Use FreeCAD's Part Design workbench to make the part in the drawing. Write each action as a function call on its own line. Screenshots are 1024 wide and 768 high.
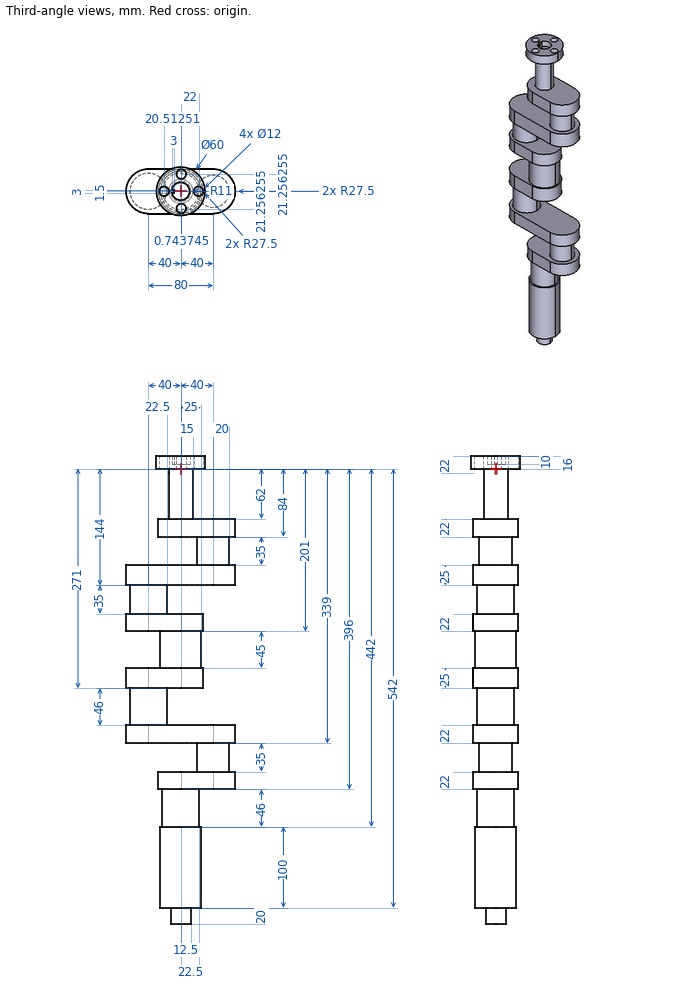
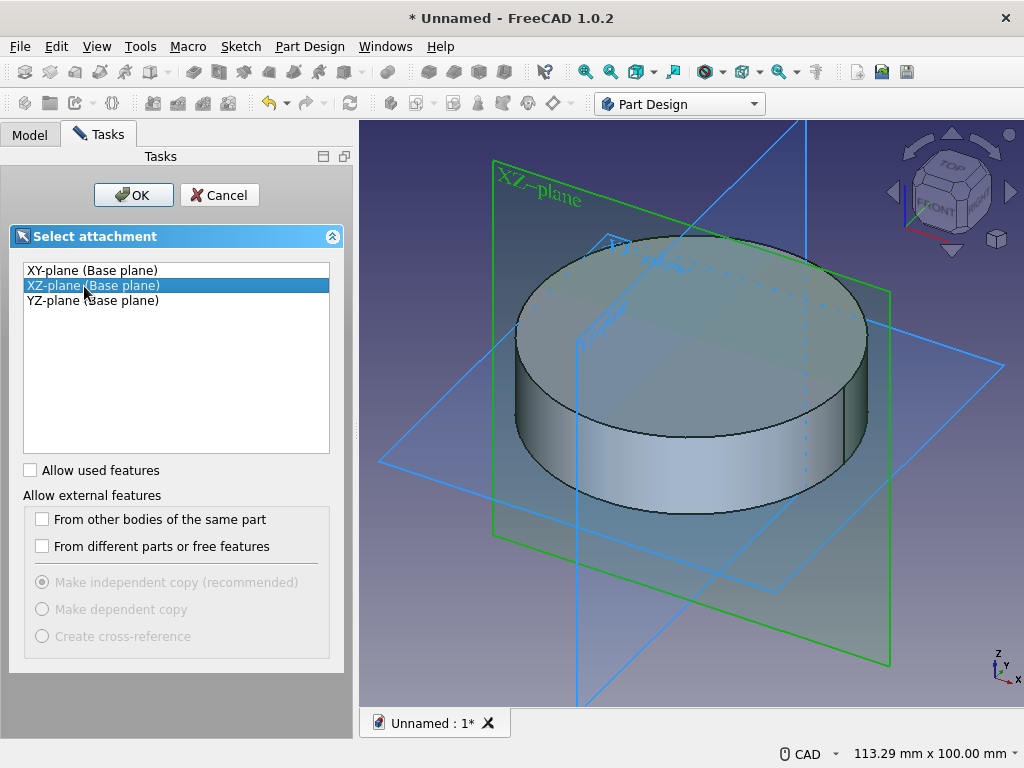
click(134, 195)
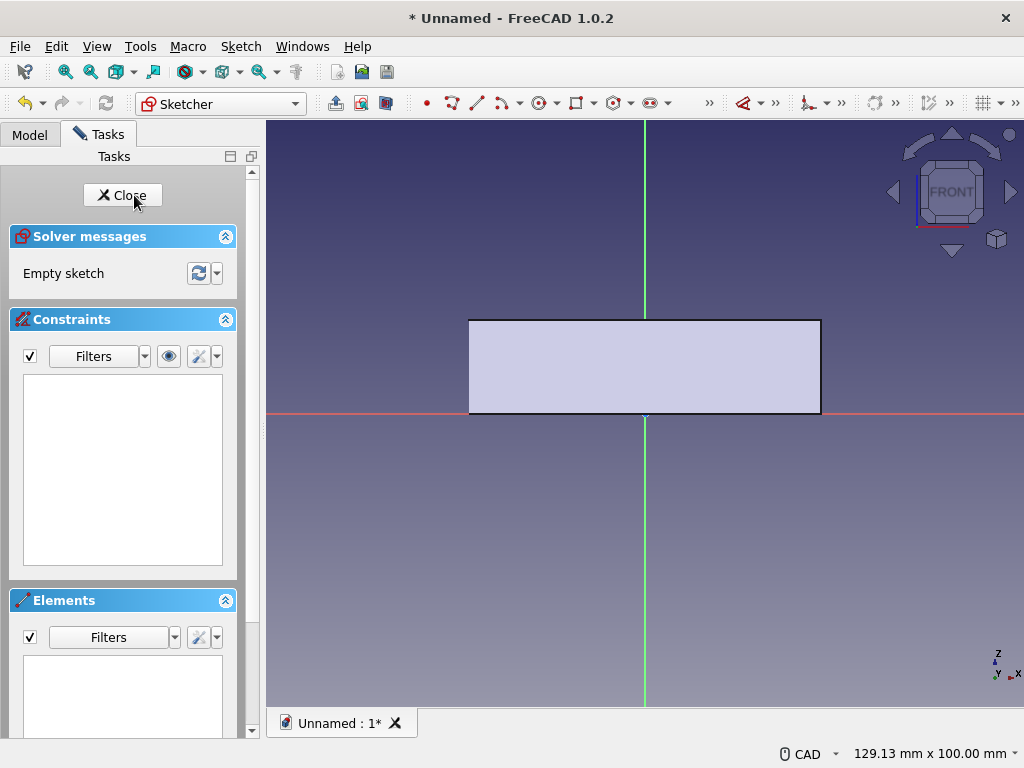
key(q)
key(s)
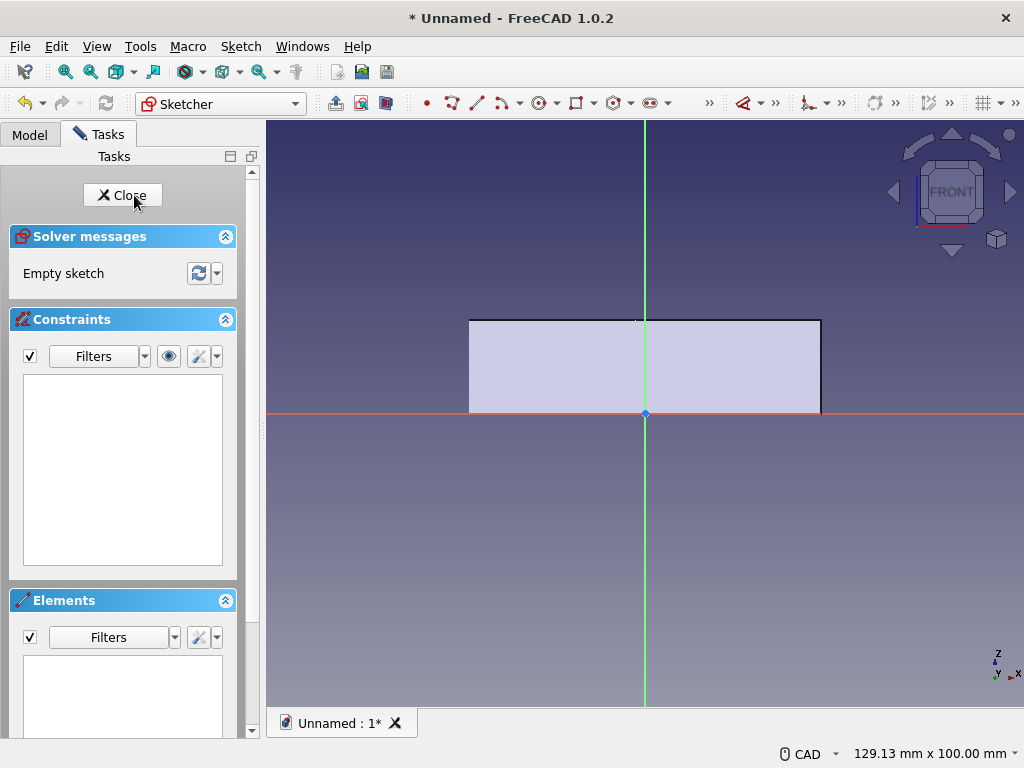
scroll(348, 148, down, 2)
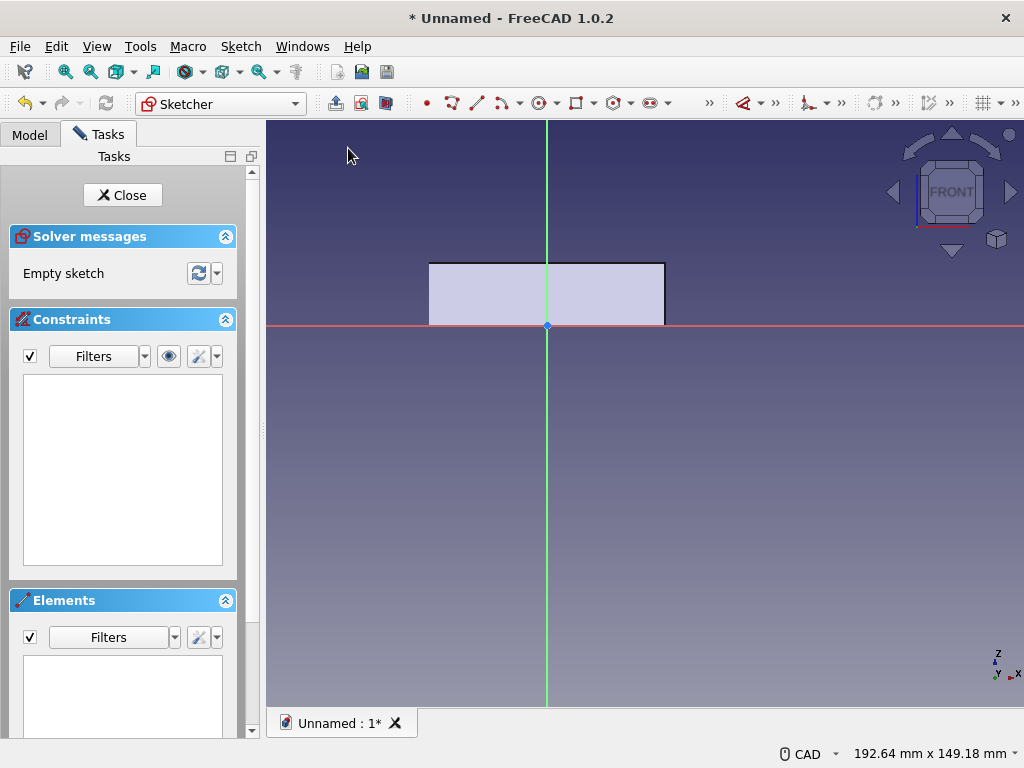
scroll(577, 518, up, 2)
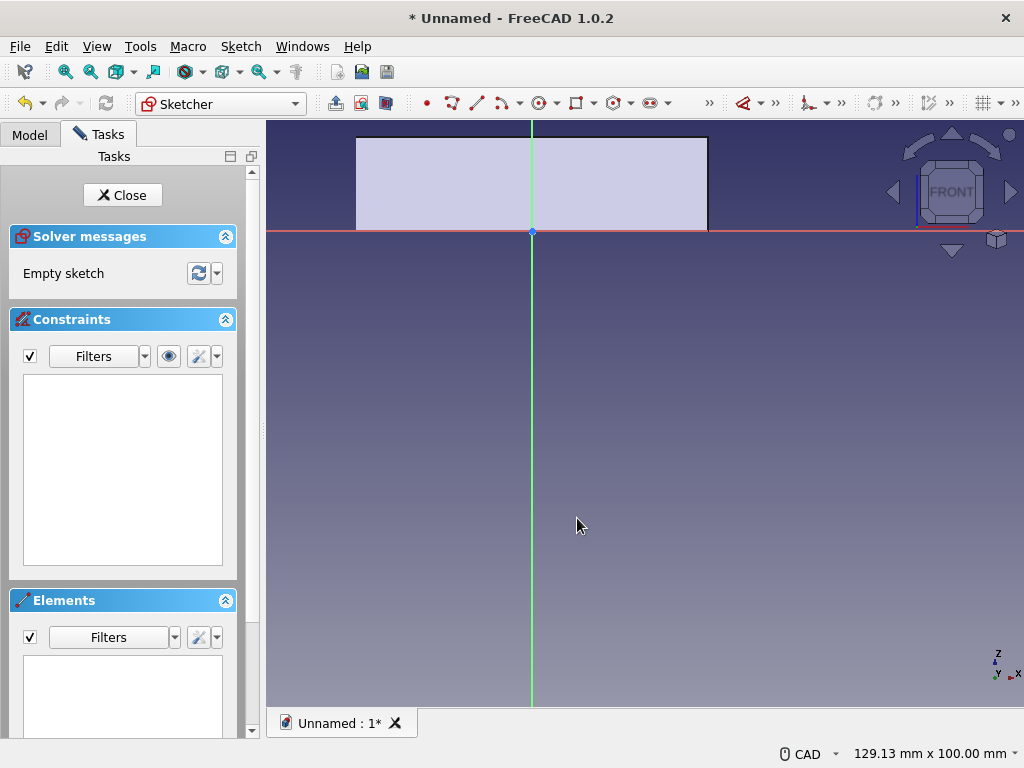
click(576, 104)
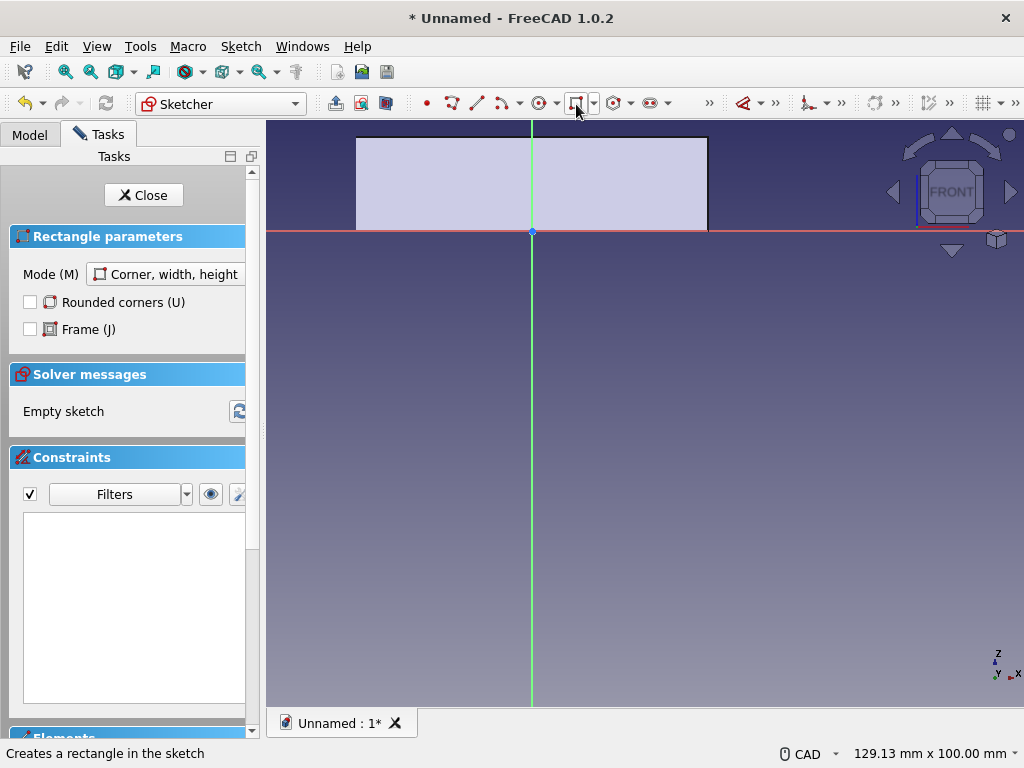
click(532, 231)
move(620, 595)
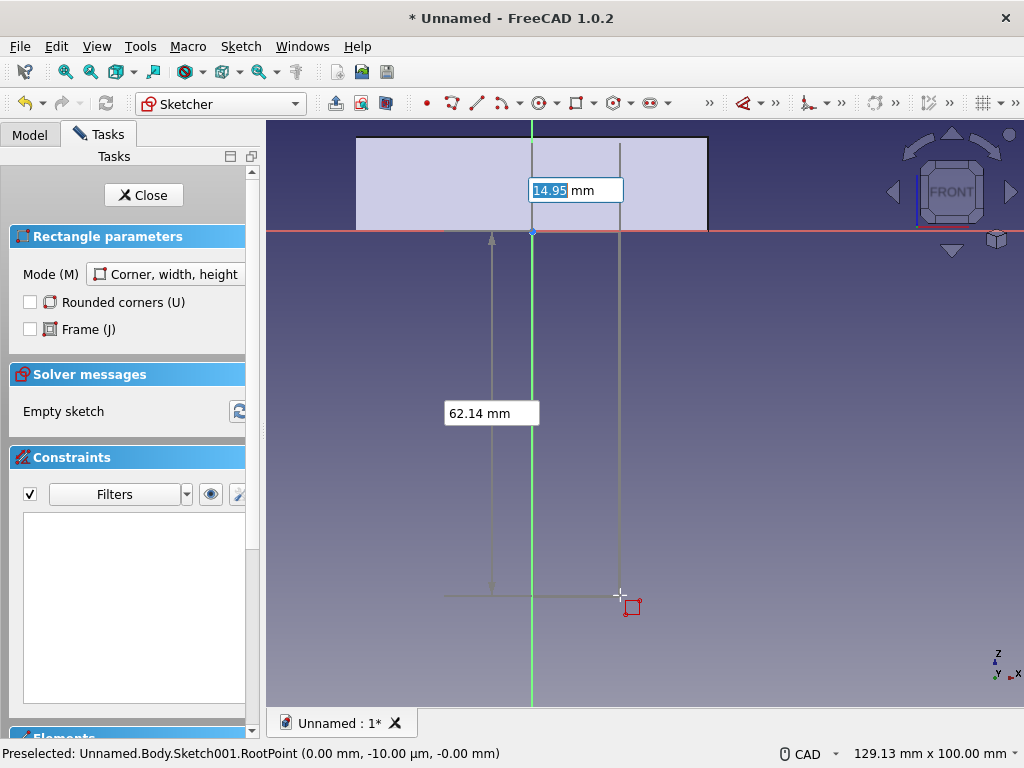
text(15)
key(Tab)
text(62)
key(Return)
key(Escape)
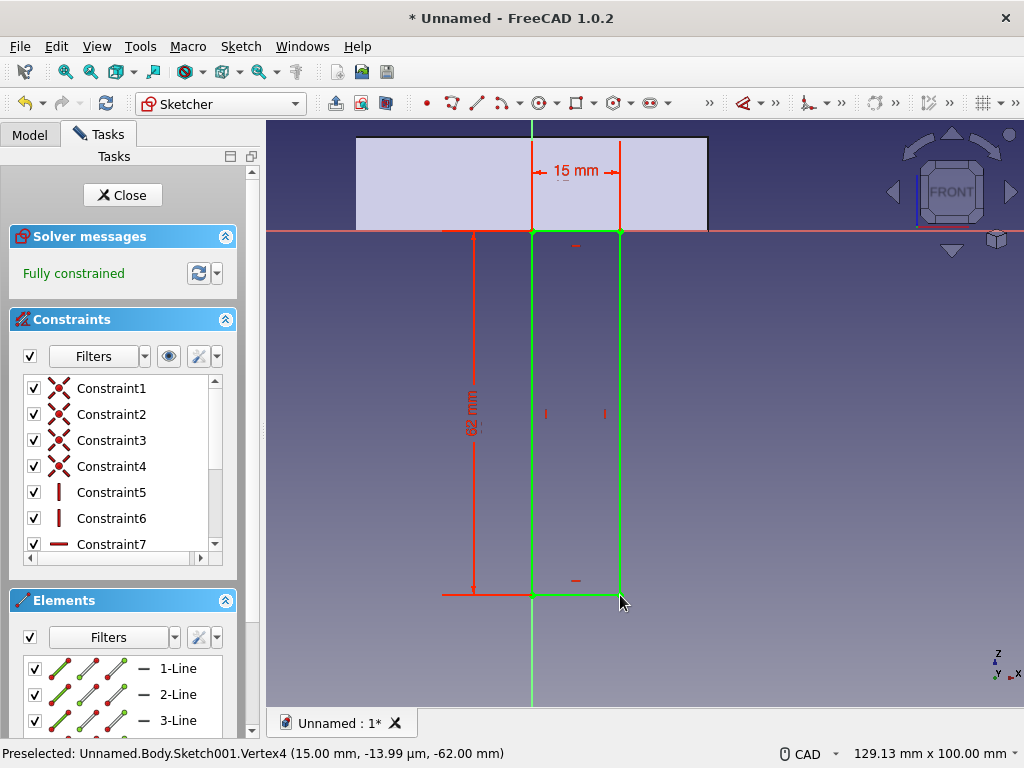
click(123, 195)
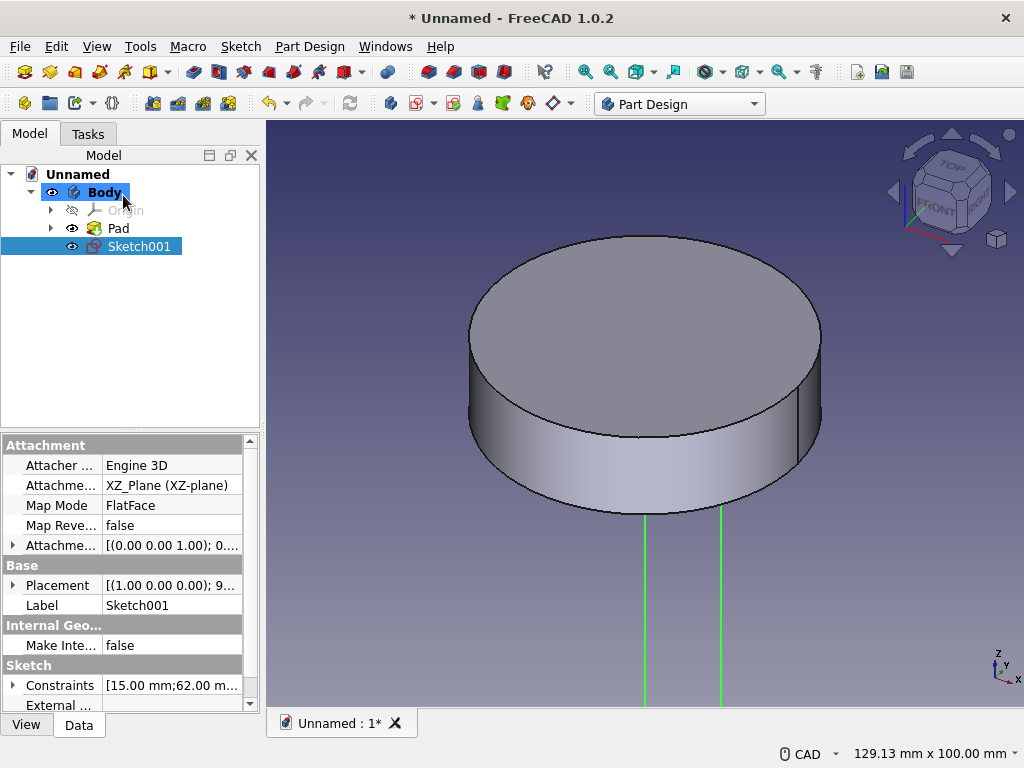
click(50, 72)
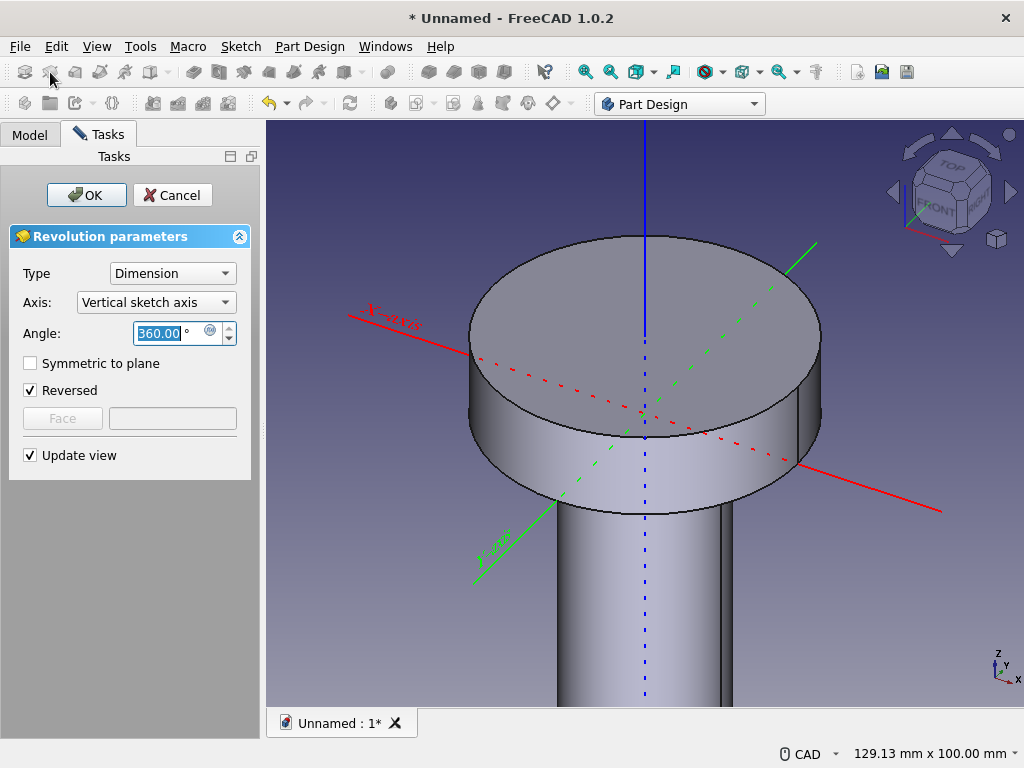
click(87, 195)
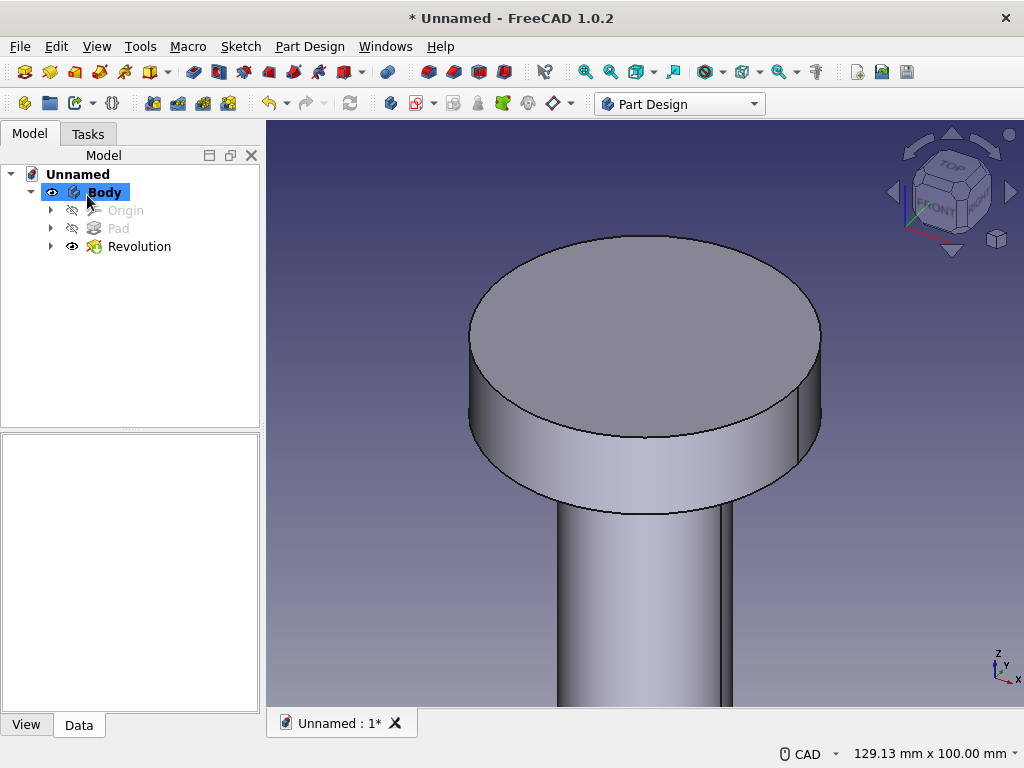
key(v)
key(f)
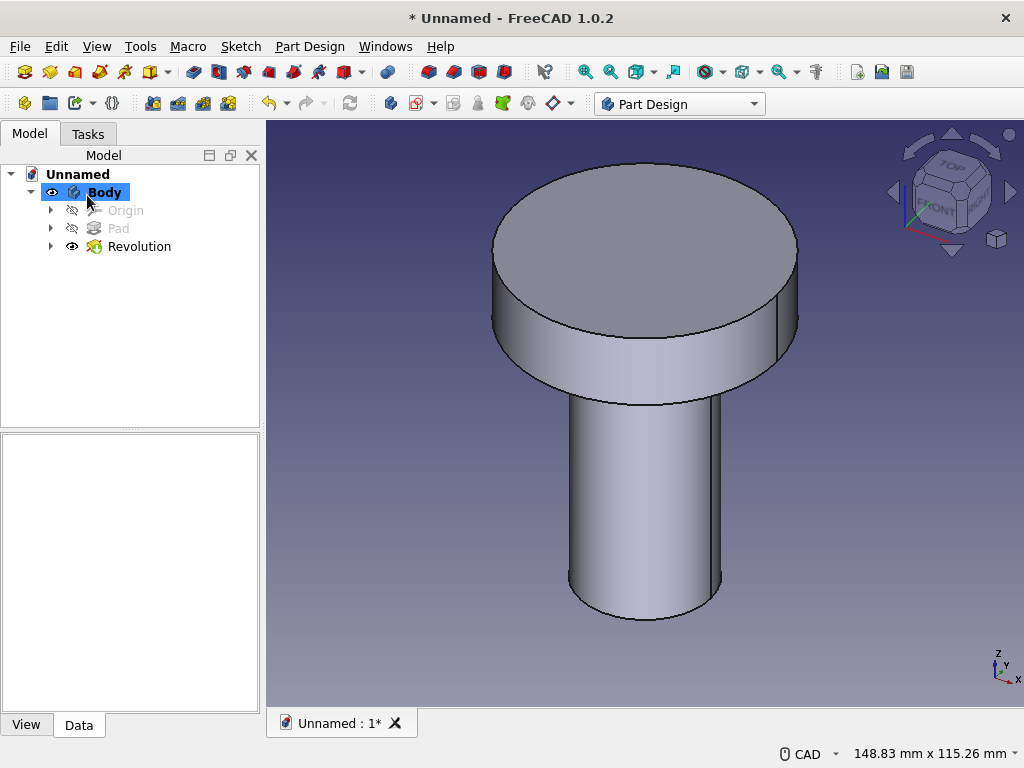
key(5)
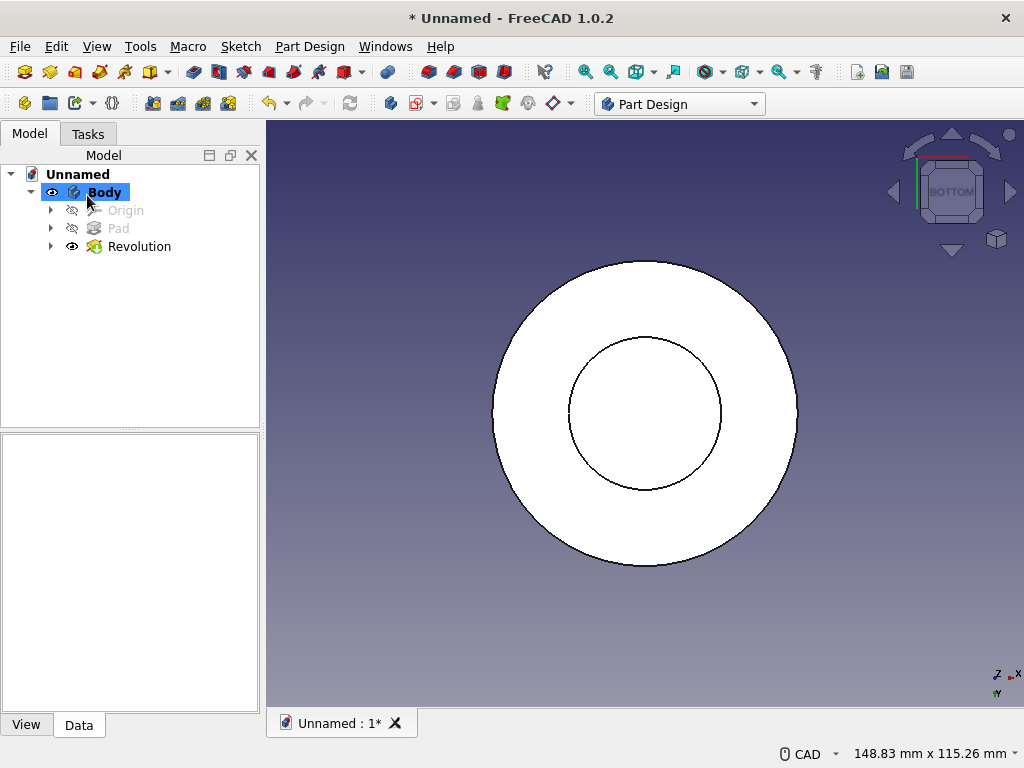
click(645, 412)